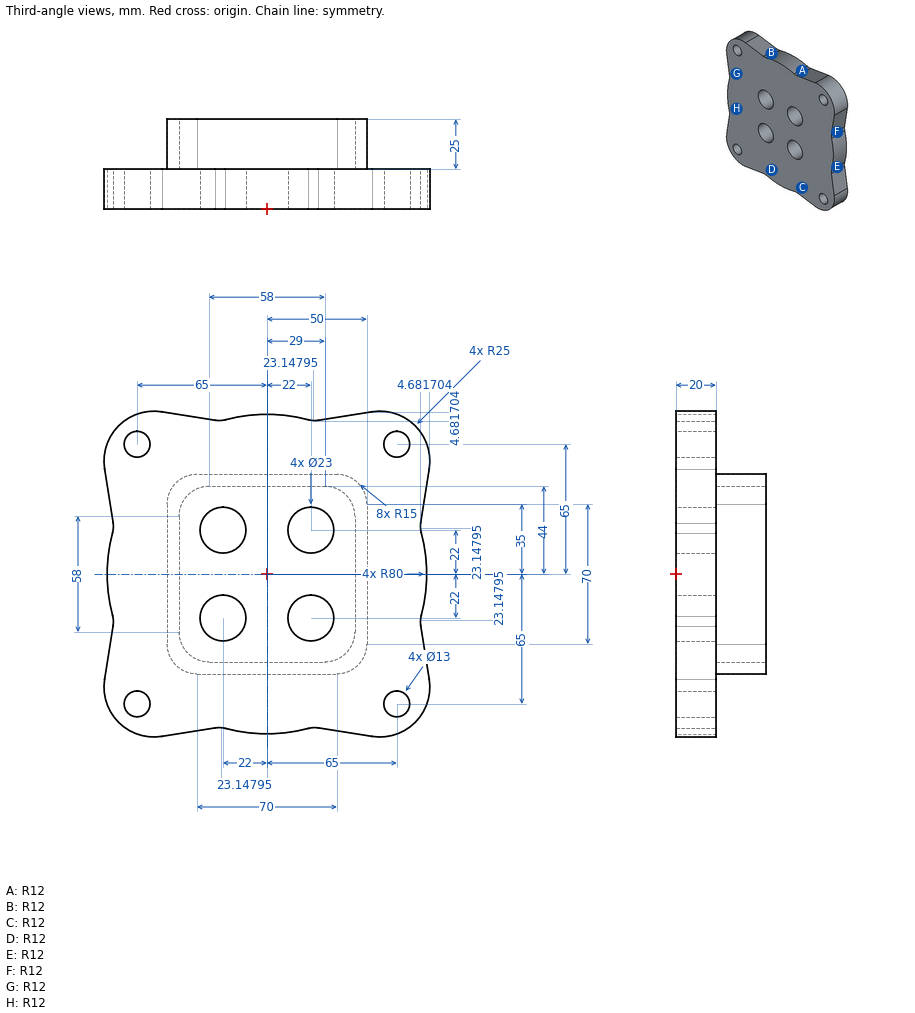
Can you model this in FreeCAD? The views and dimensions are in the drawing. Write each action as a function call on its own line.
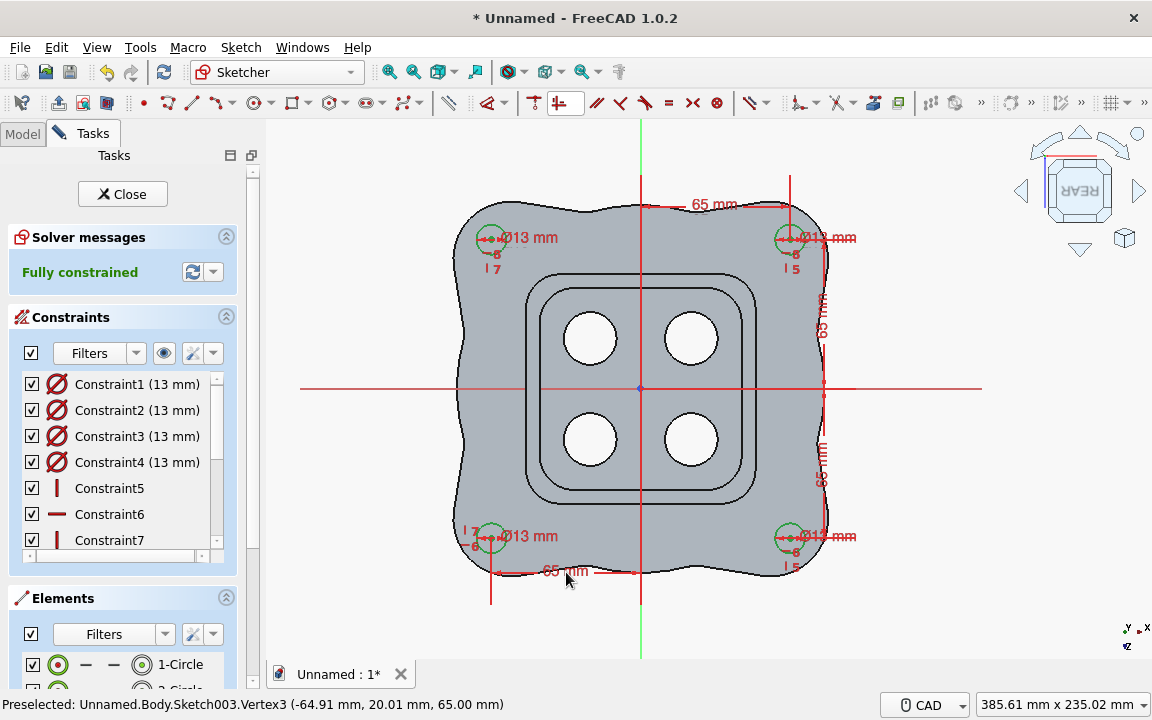
click(123, 194)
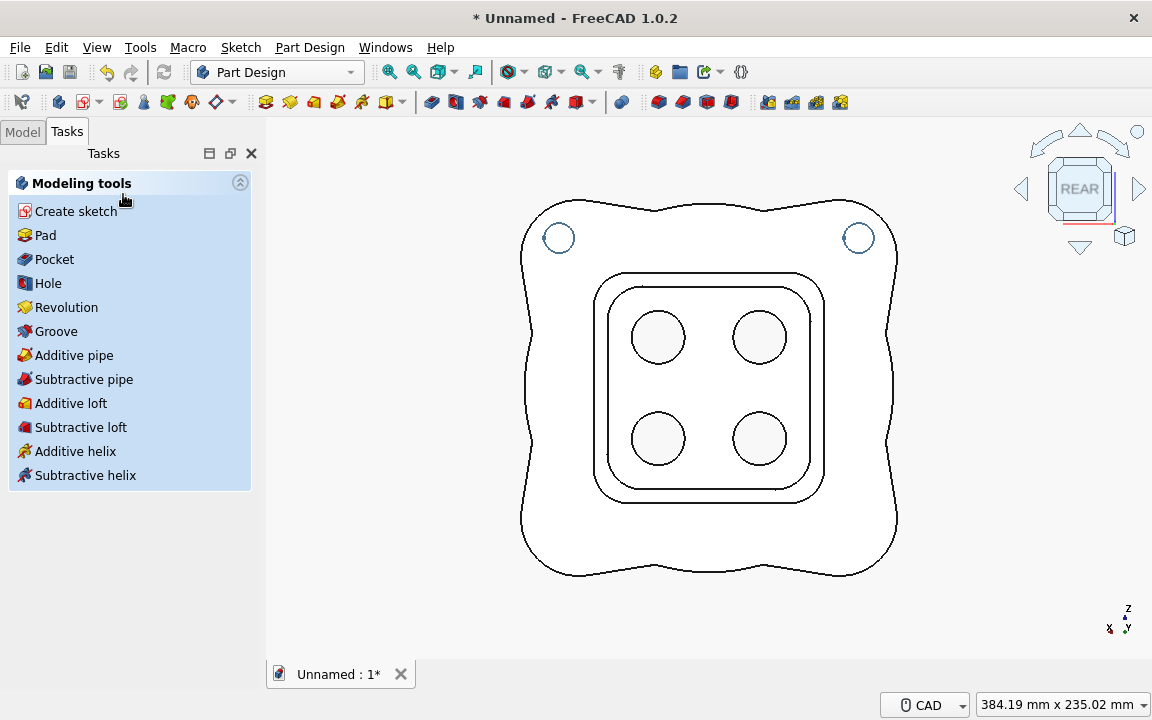
click(432, 102)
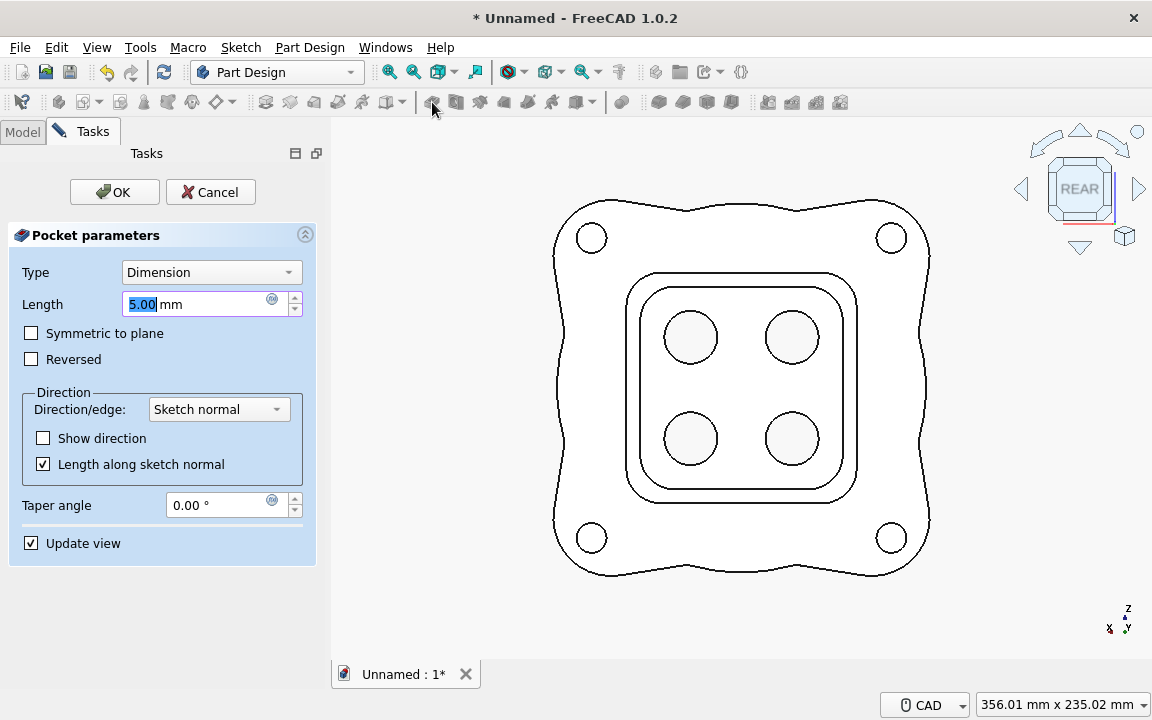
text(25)
key(Tab)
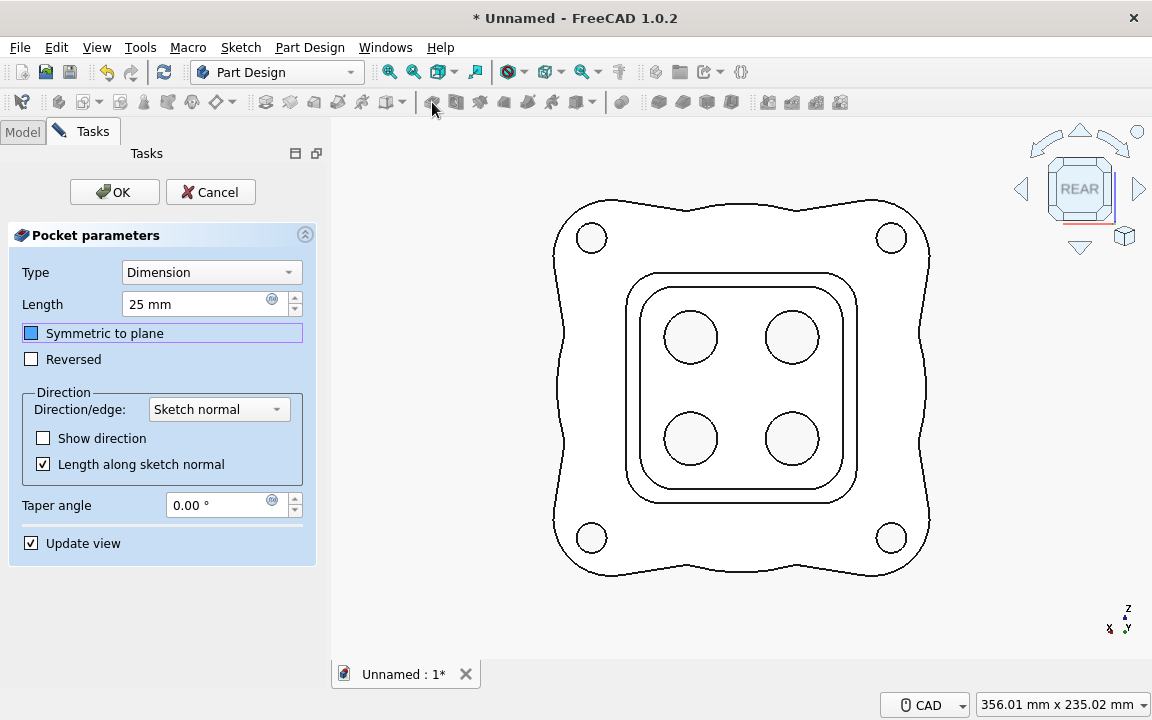
click(115, 192)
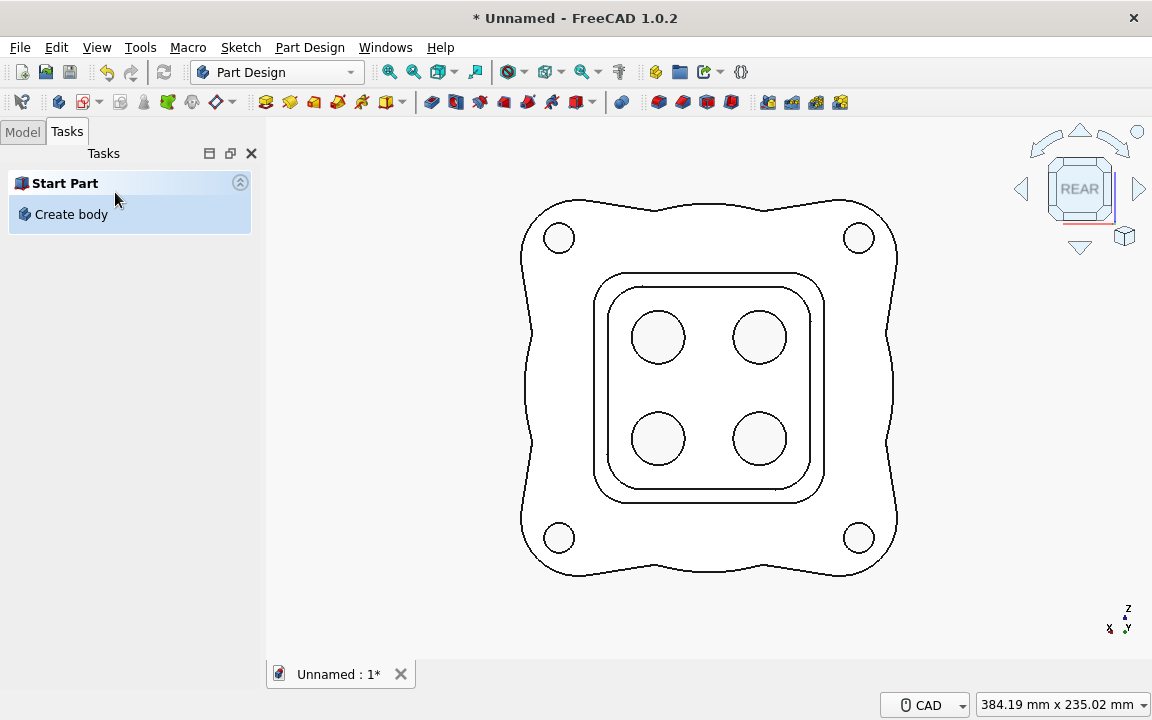
key(0)